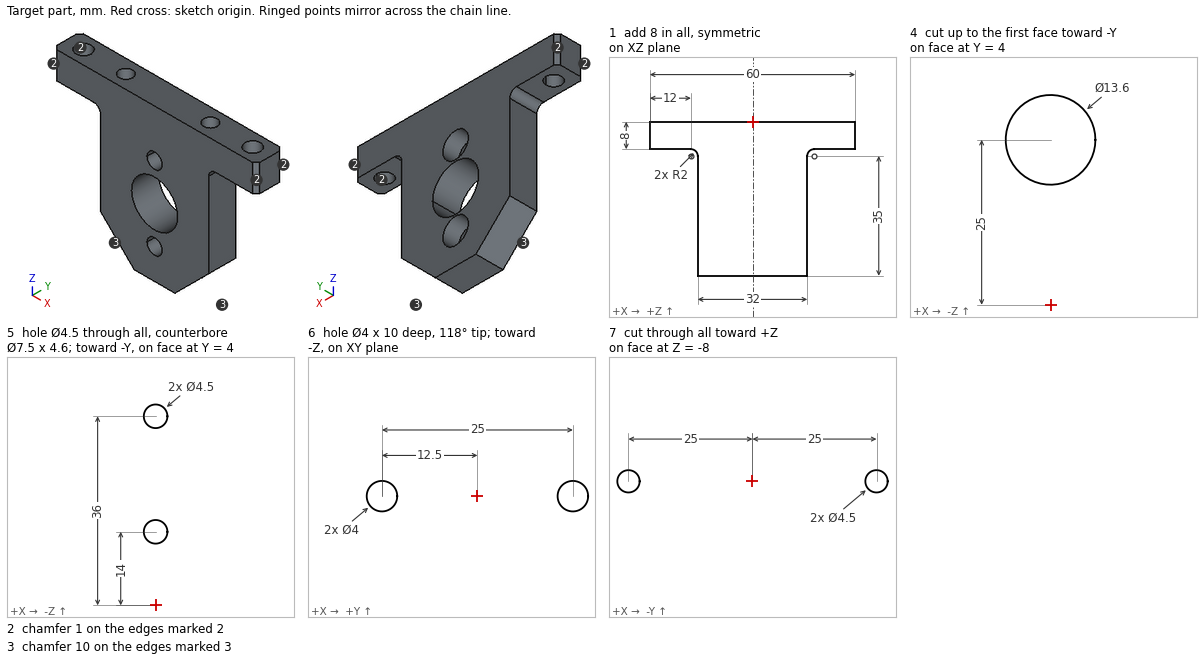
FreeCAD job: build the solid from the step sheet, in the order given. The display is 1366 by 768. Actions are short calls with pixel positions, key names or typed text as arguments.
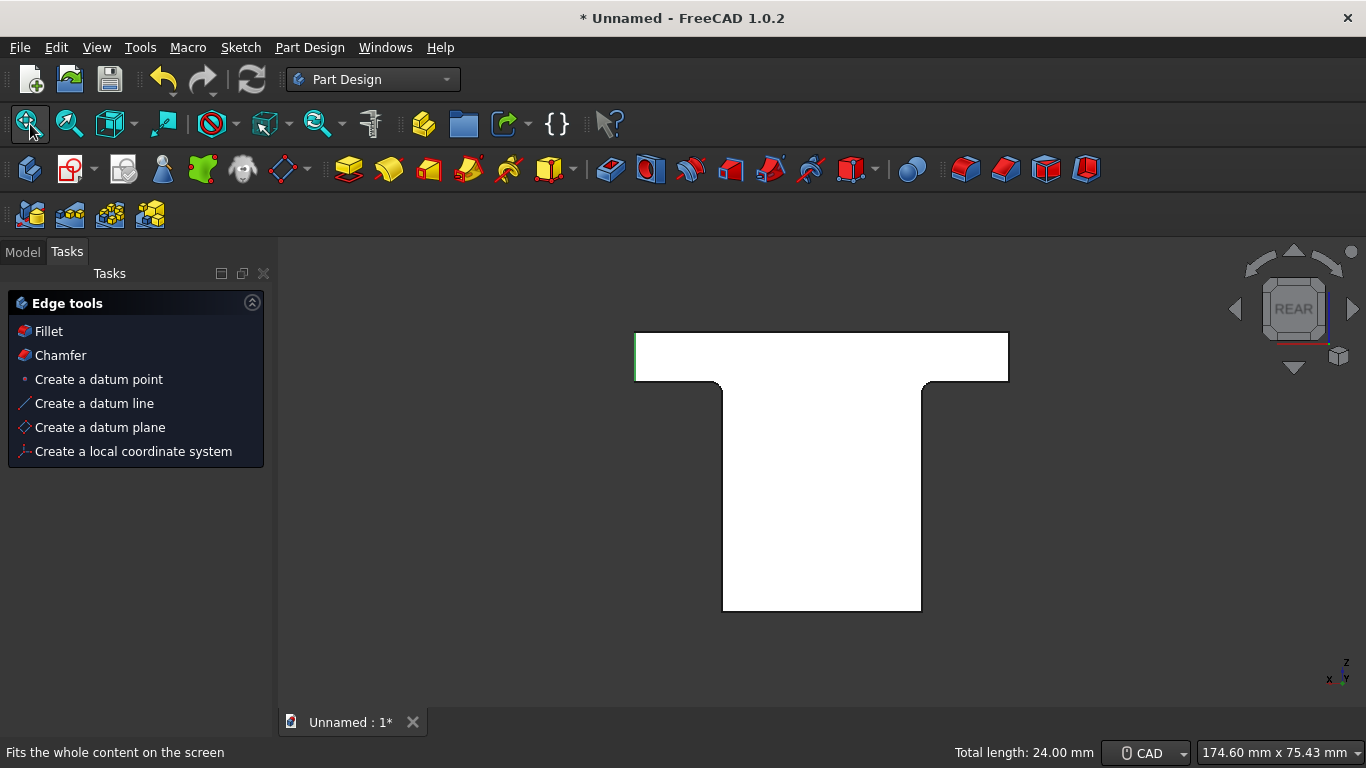
click(1009, 356, ctrl)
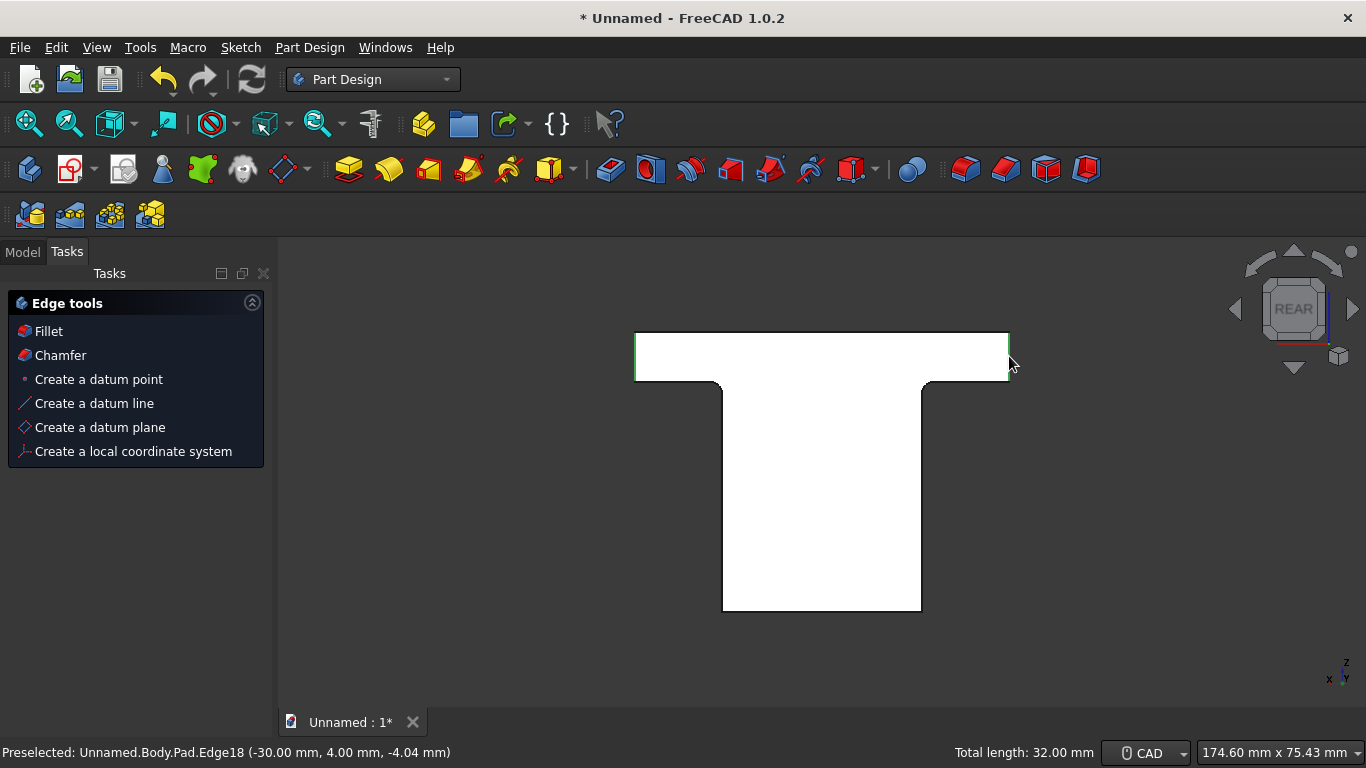
click(1006, 170)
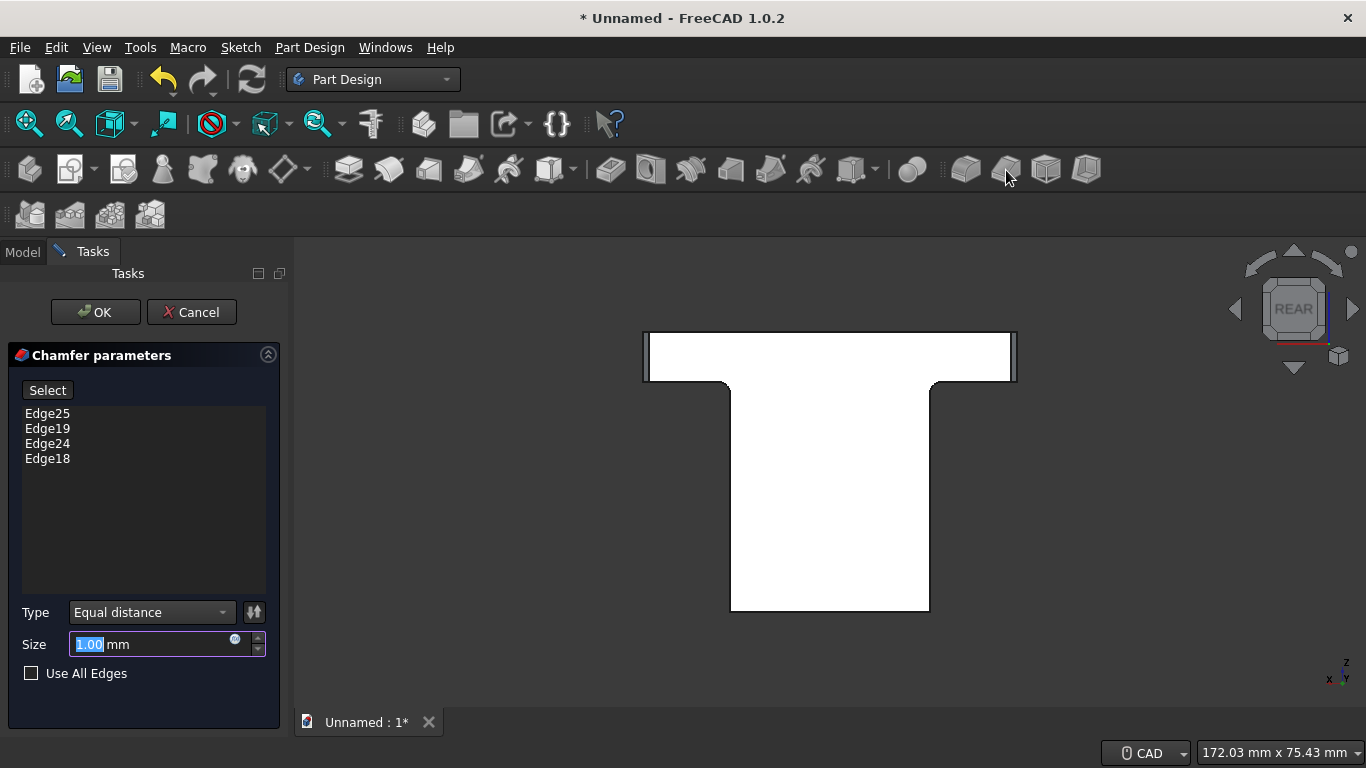
text(1)
key(Tab)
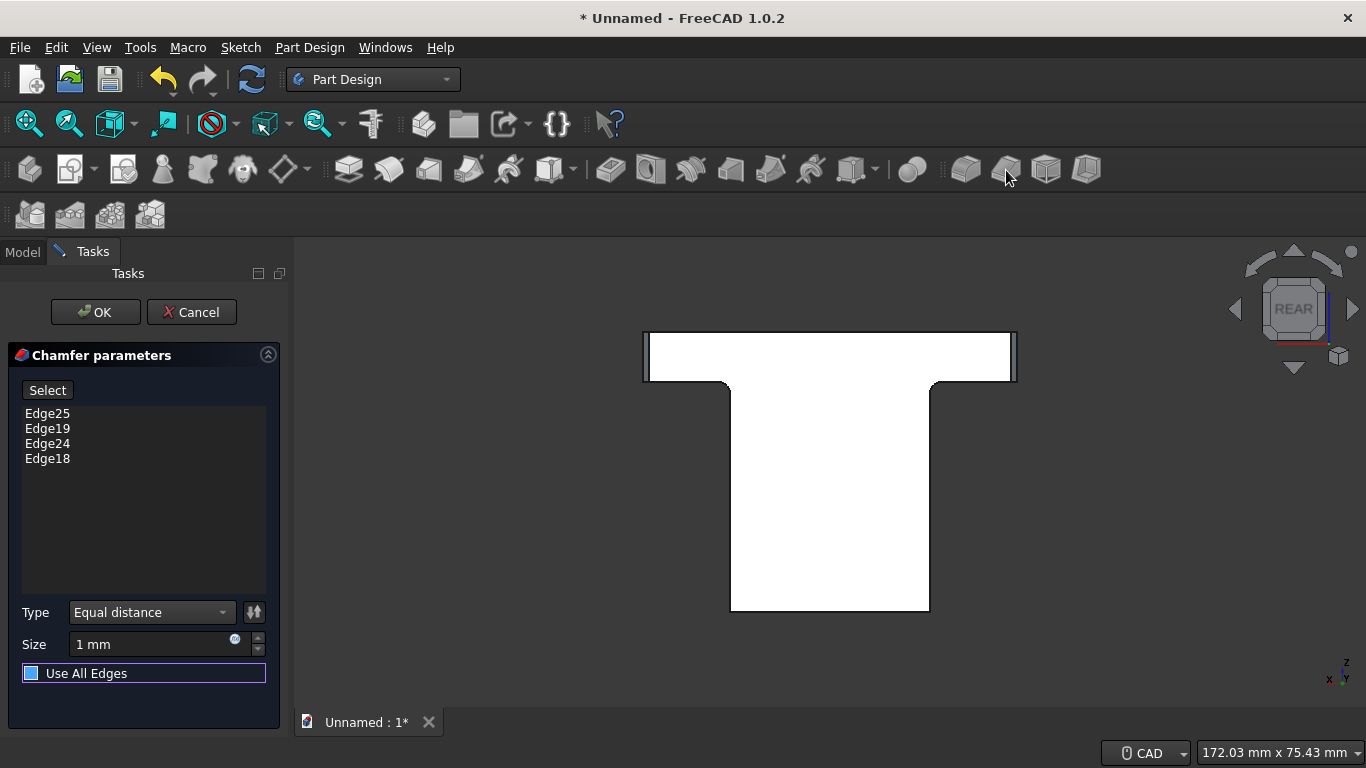
click(96, 312)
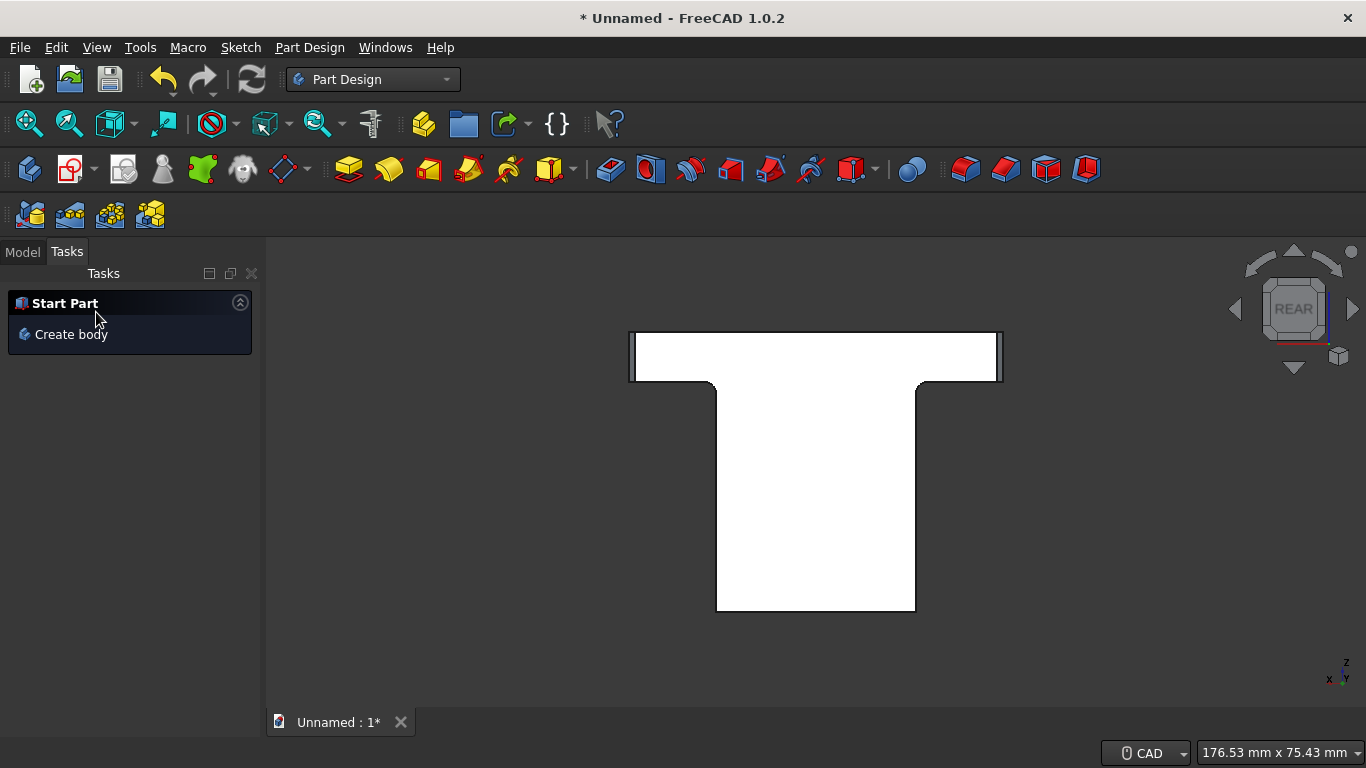
key(0)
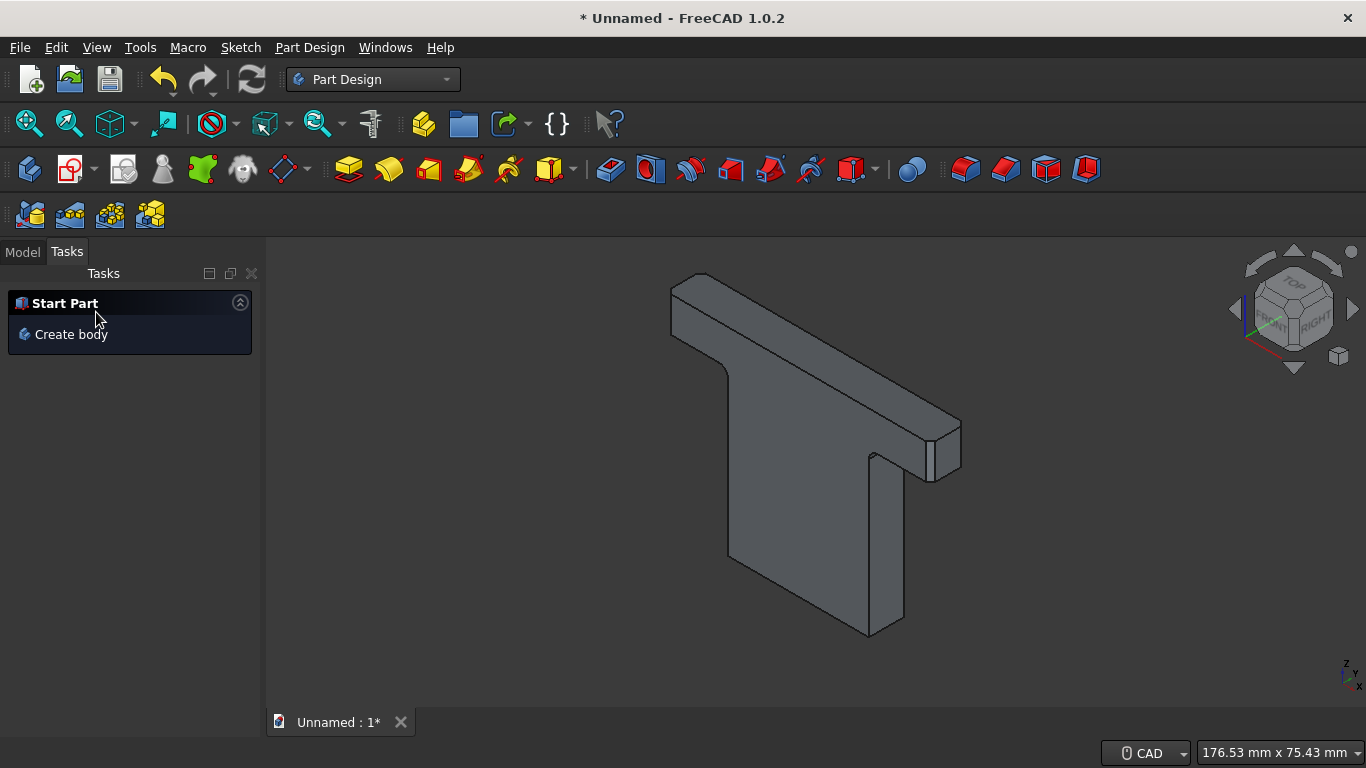
key(2)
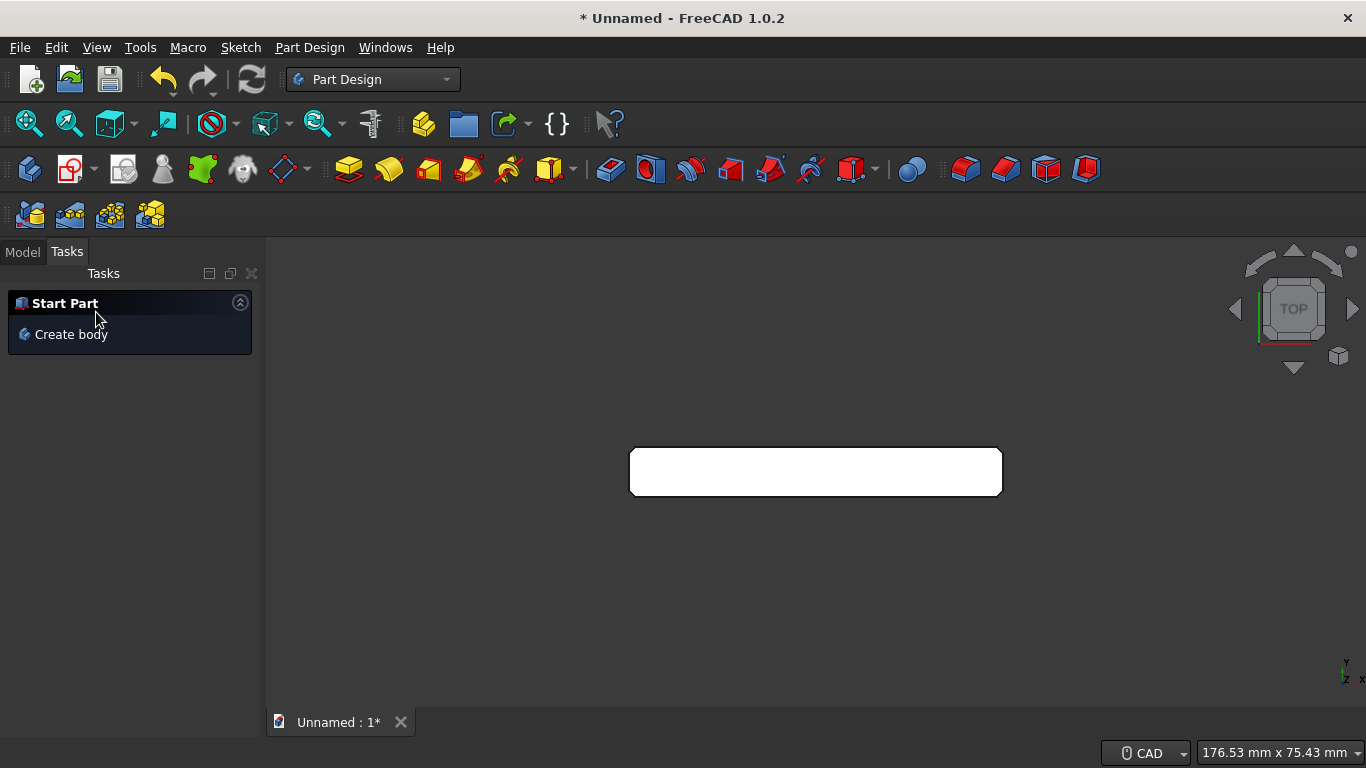
click(30, 124)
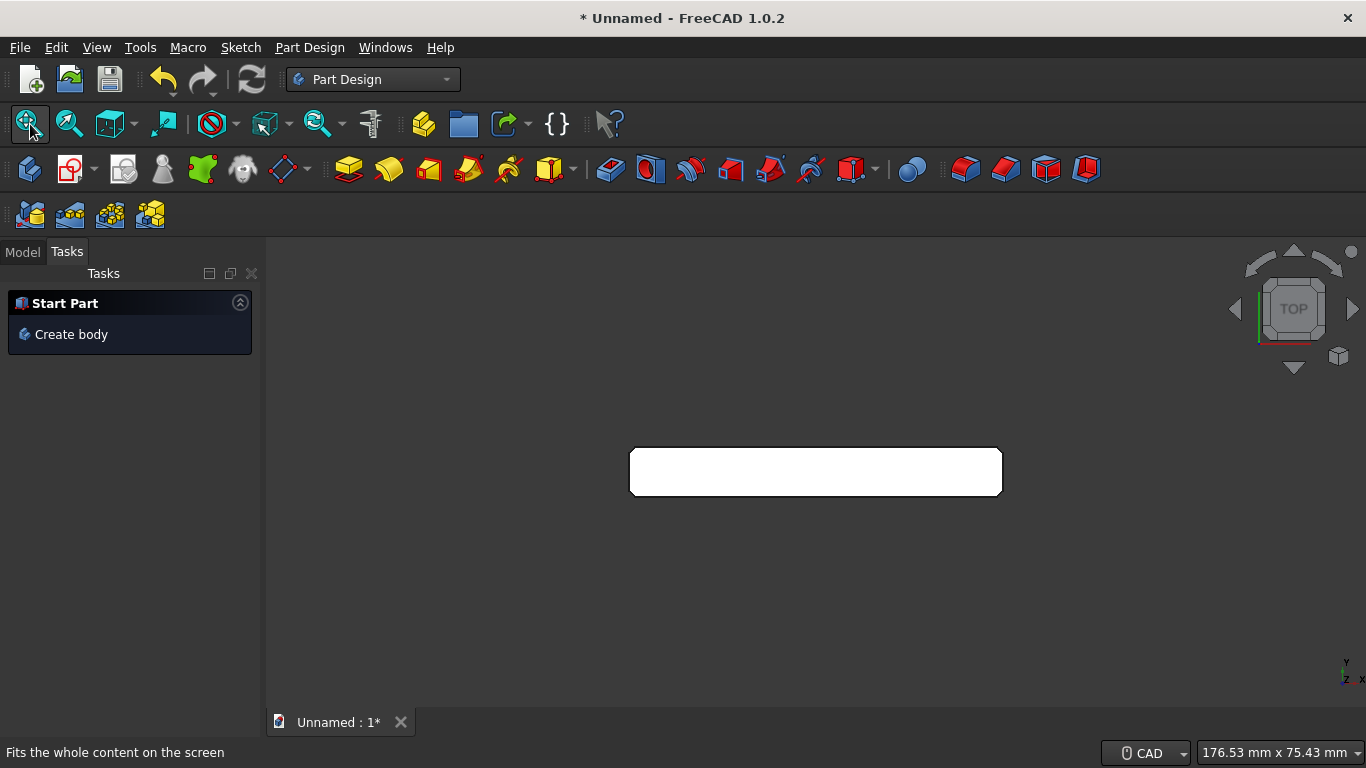
key(1)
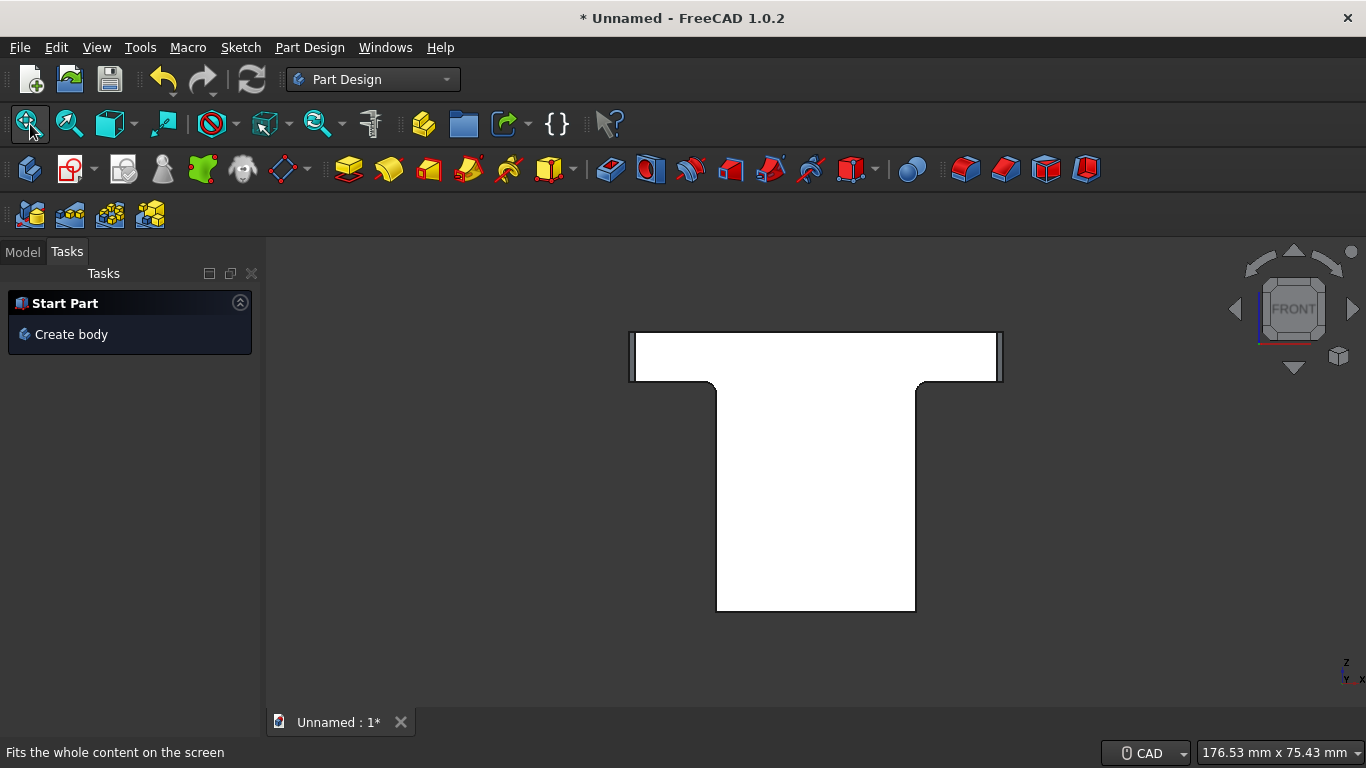
key(3)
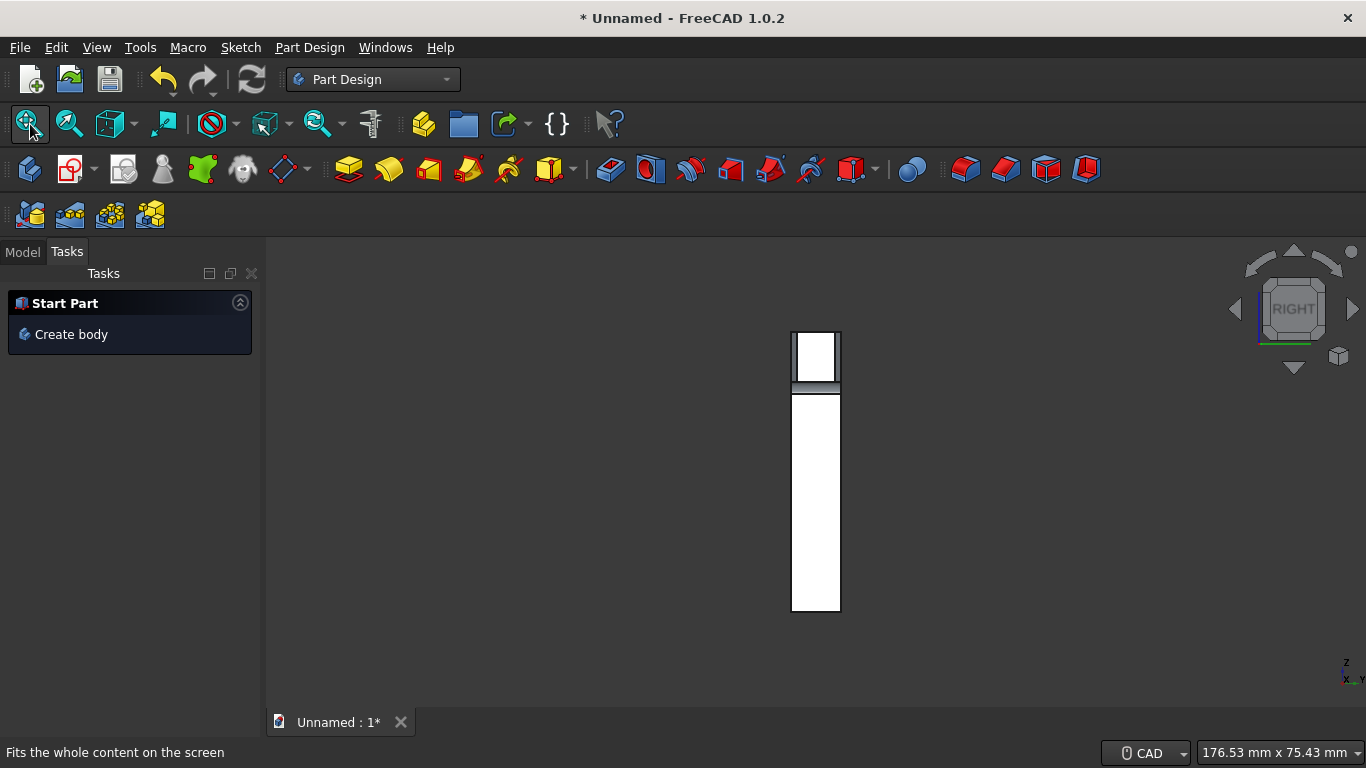
click(816, 611)